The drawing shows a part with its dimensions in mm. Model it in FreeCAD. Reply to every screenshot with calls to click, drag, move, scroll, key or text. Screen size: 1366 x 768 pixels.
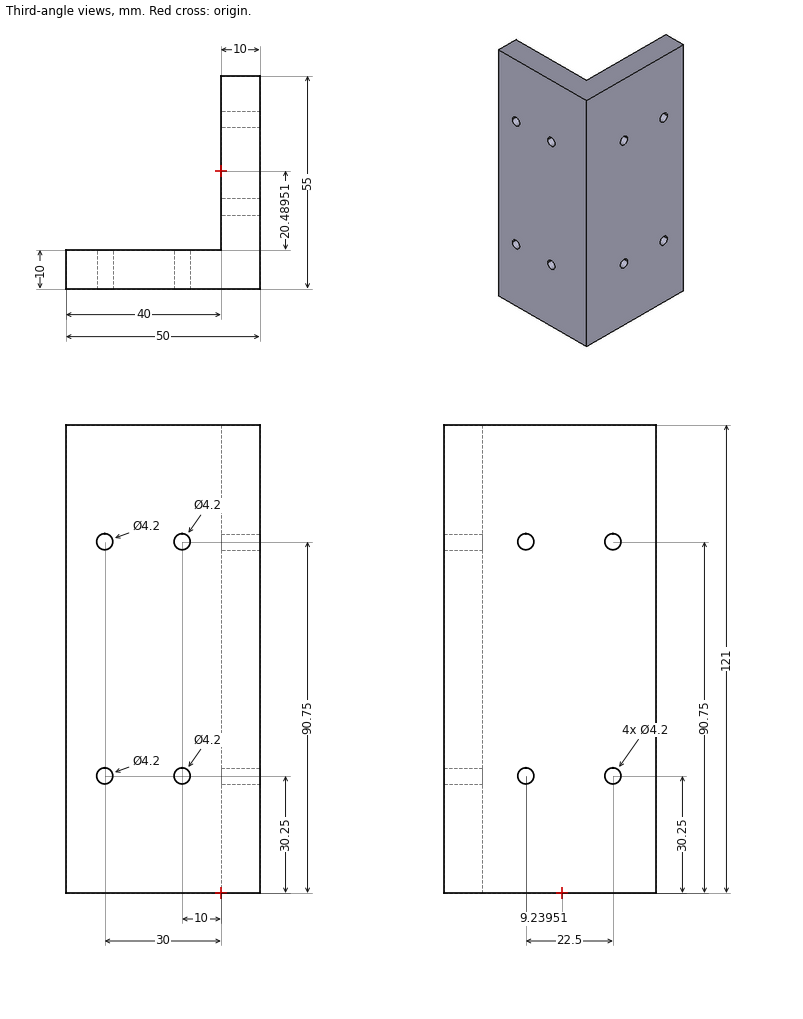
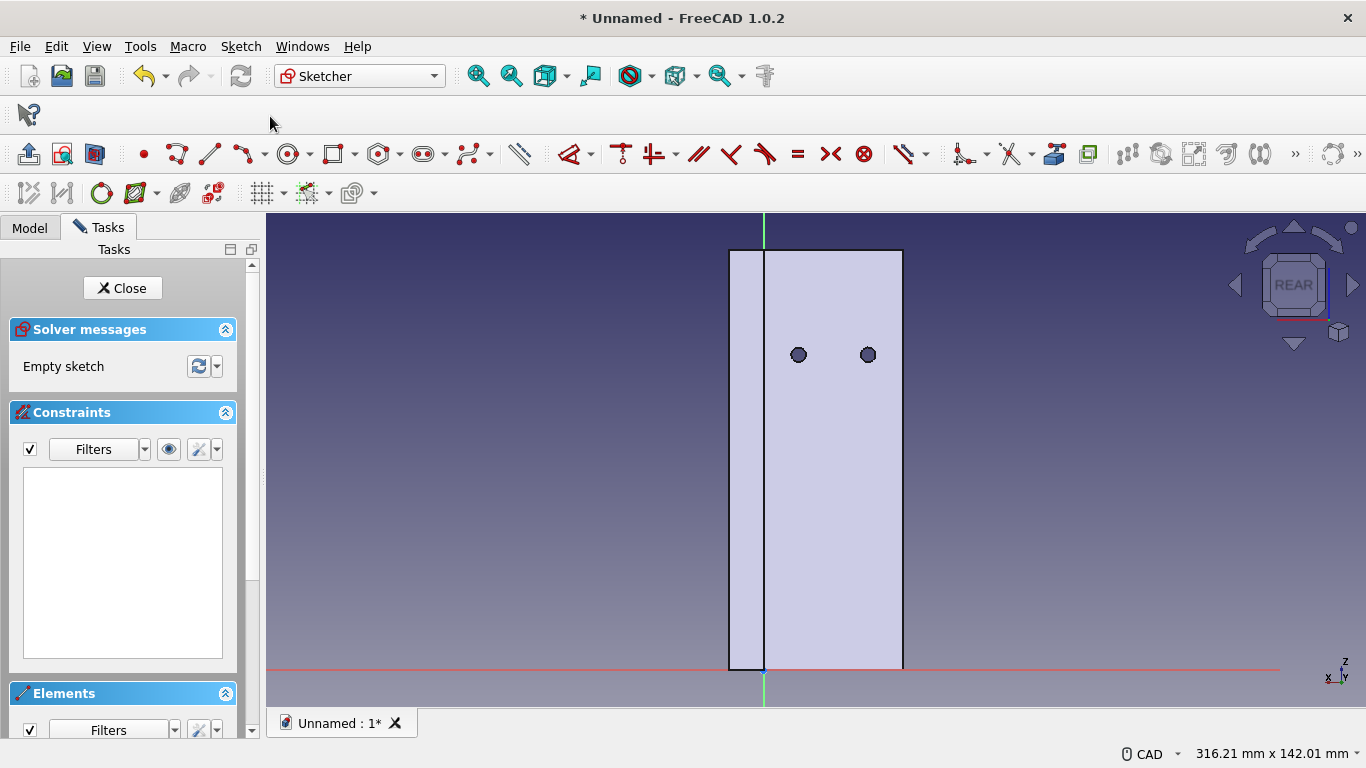
scroll(875, 571, up, 15)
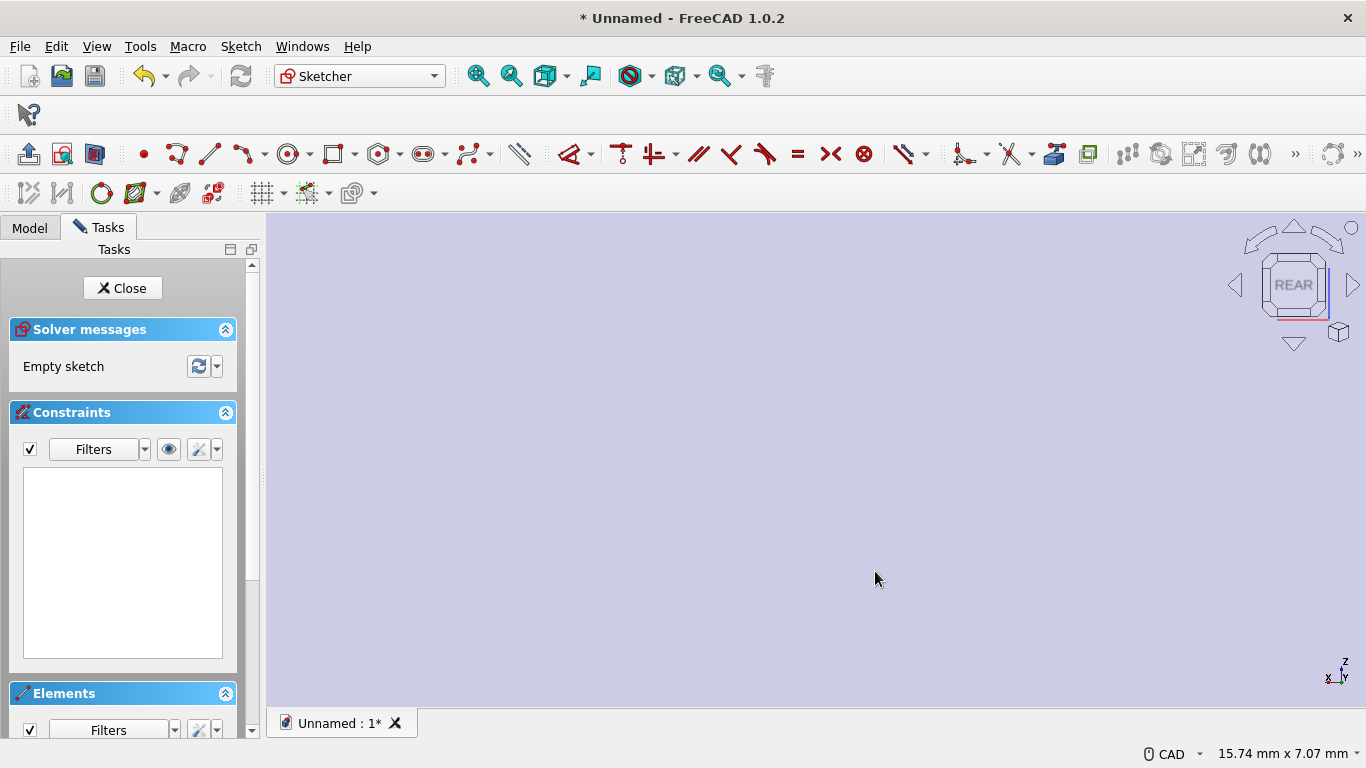
key(g)
key(c)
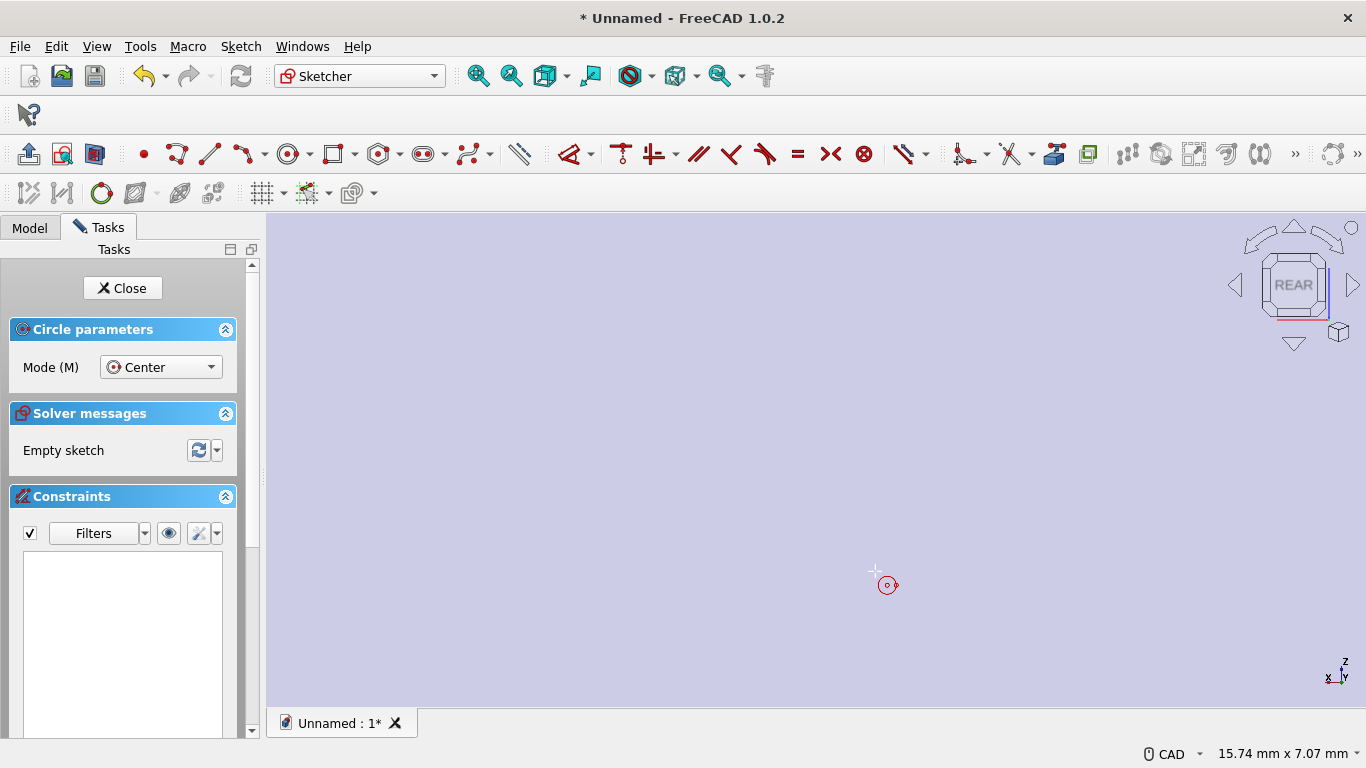
click(727, 441)
move(831, 338)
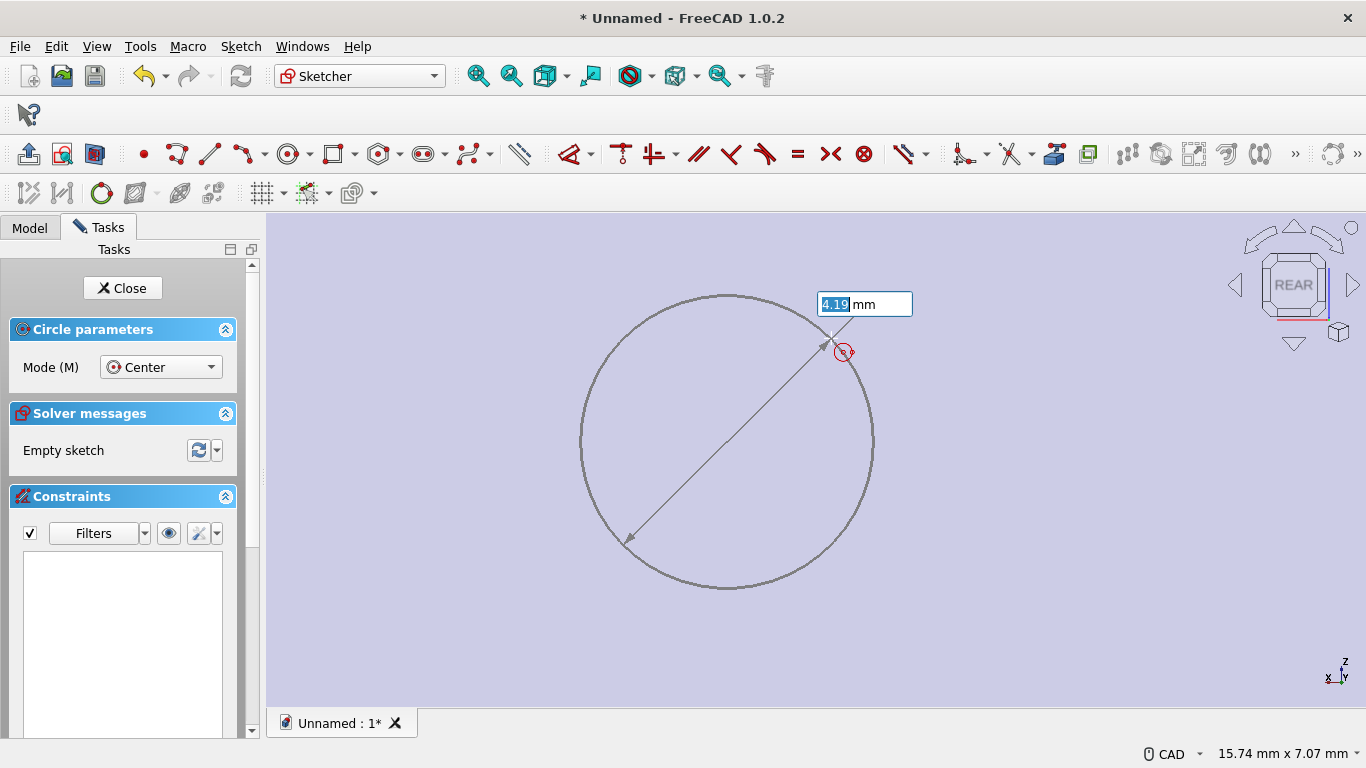
text(4.2)
key(Return)
key(Escape)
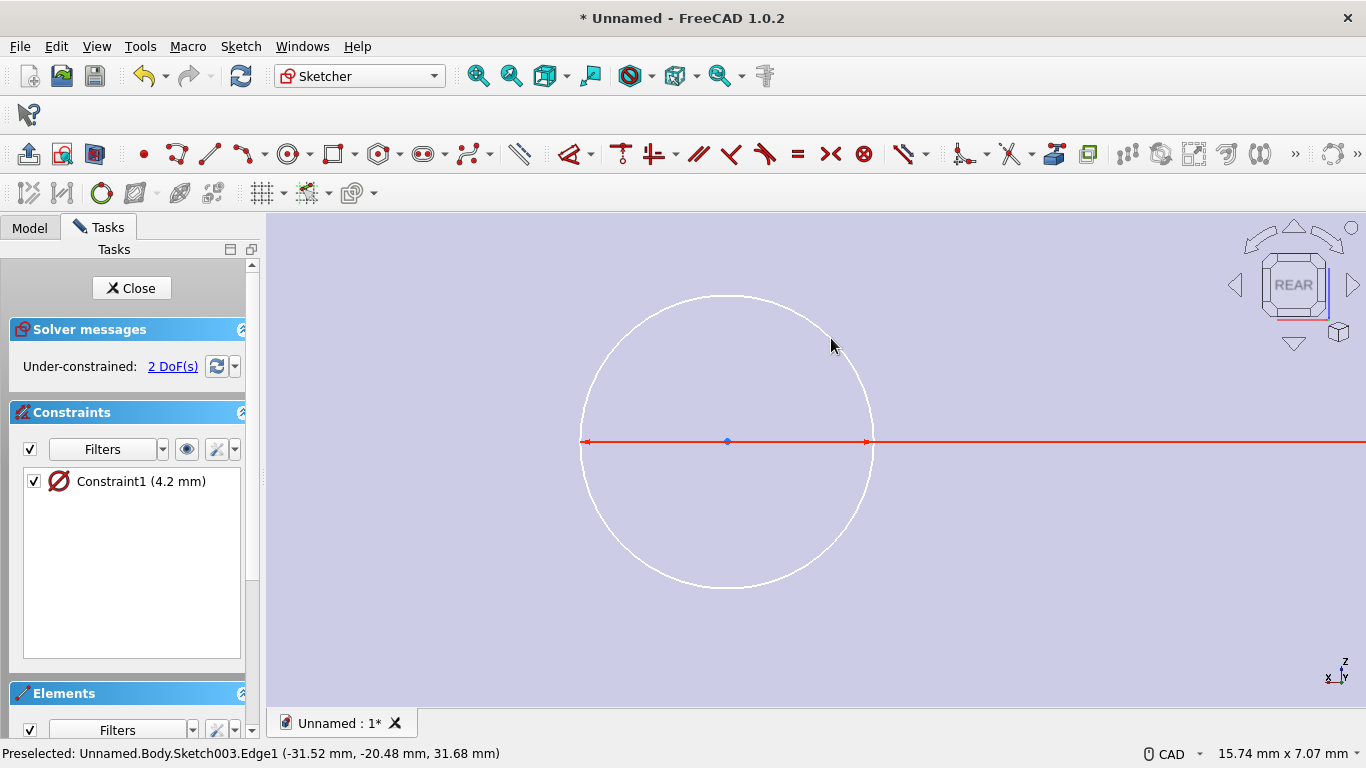
click(568, 154)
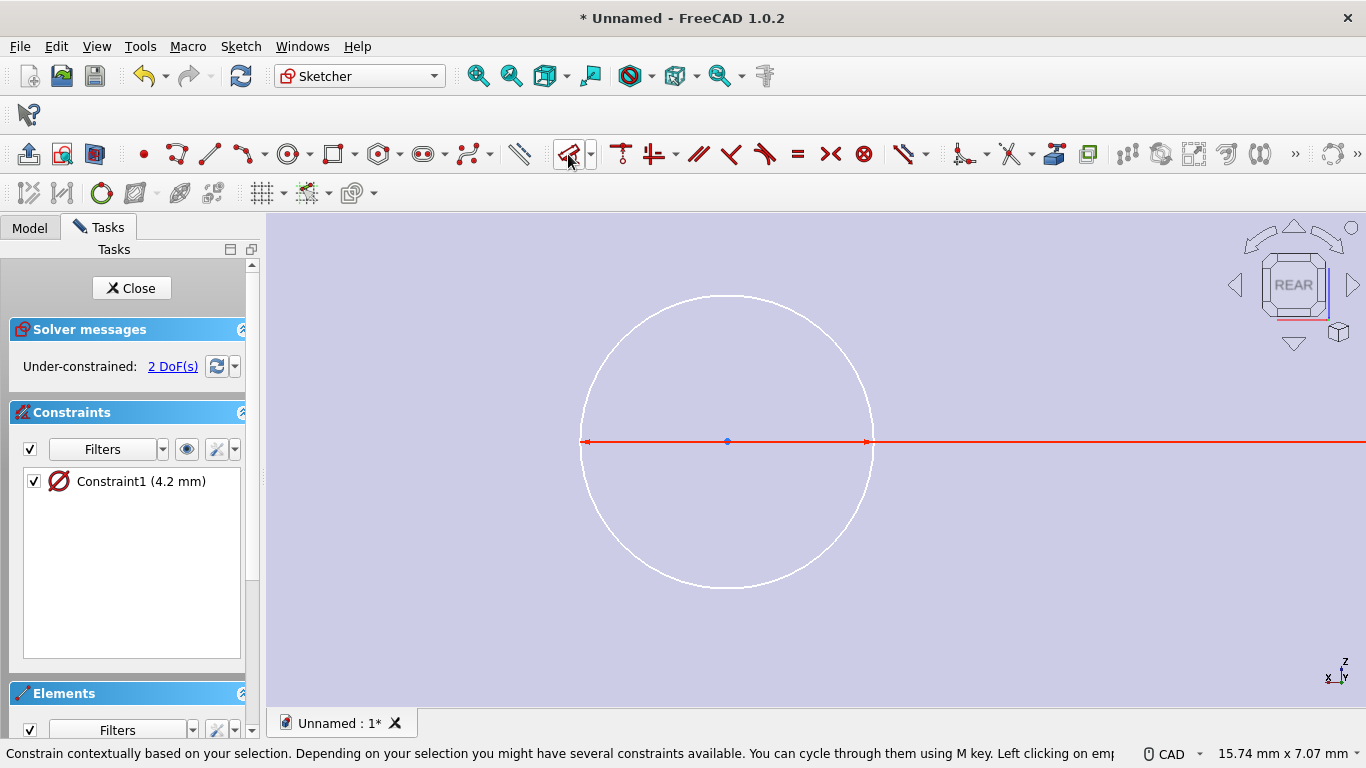
click(727, 442)
click(511, 408)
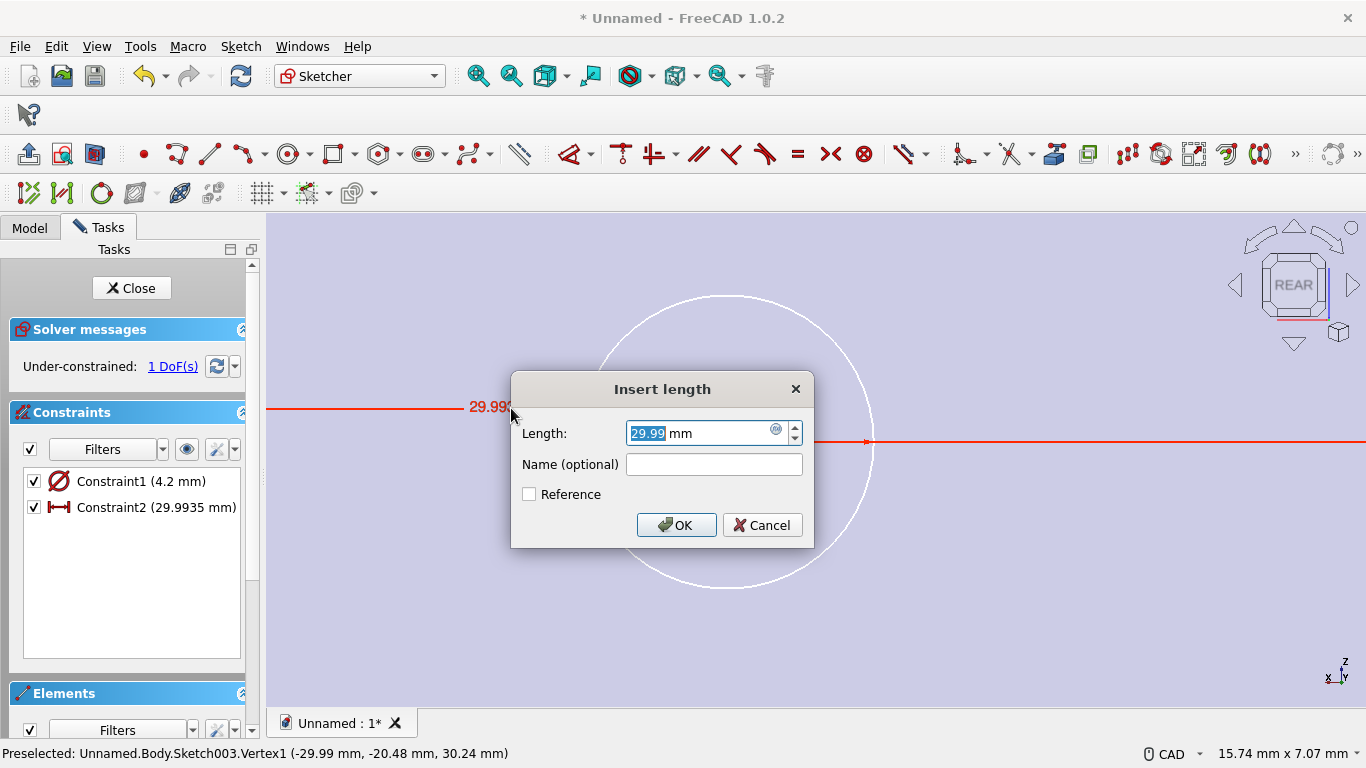
text(30)
key(Return)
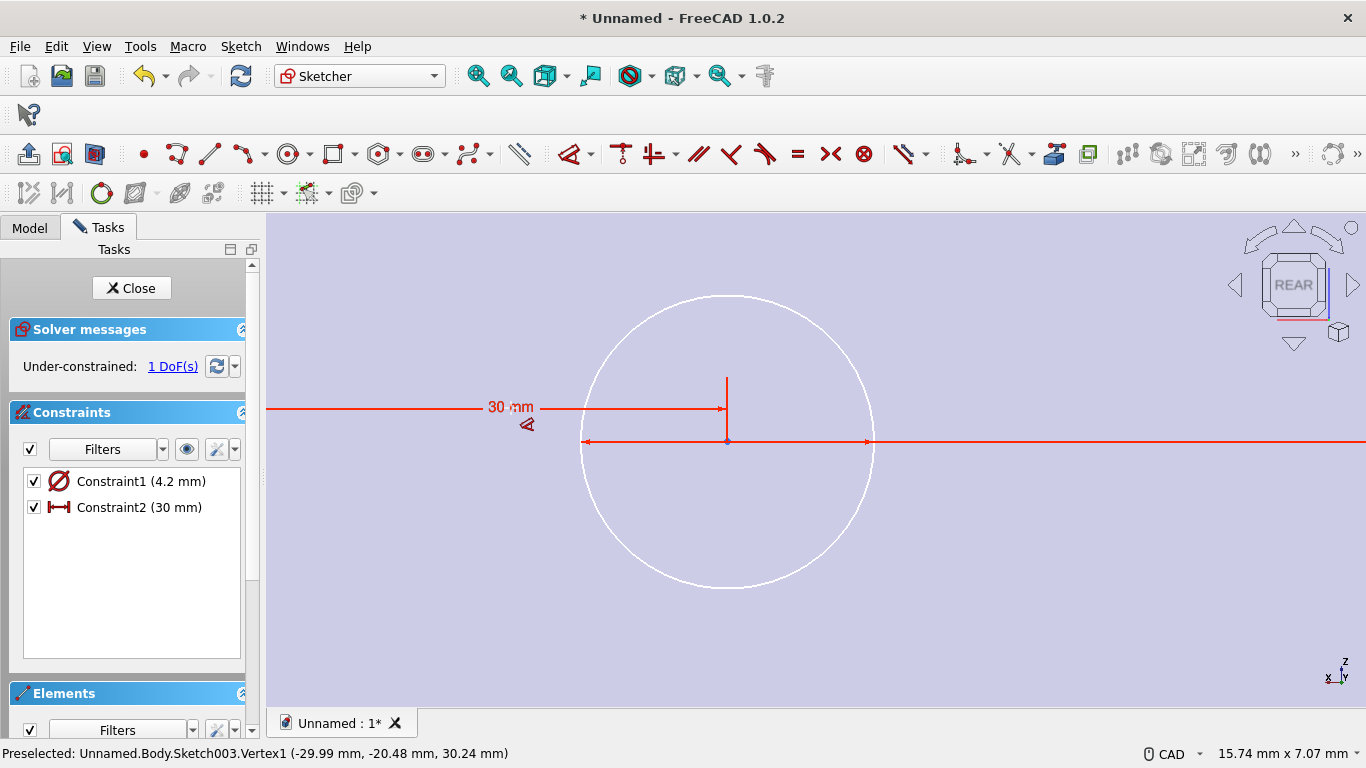
click(727, 442)
click(761, 561)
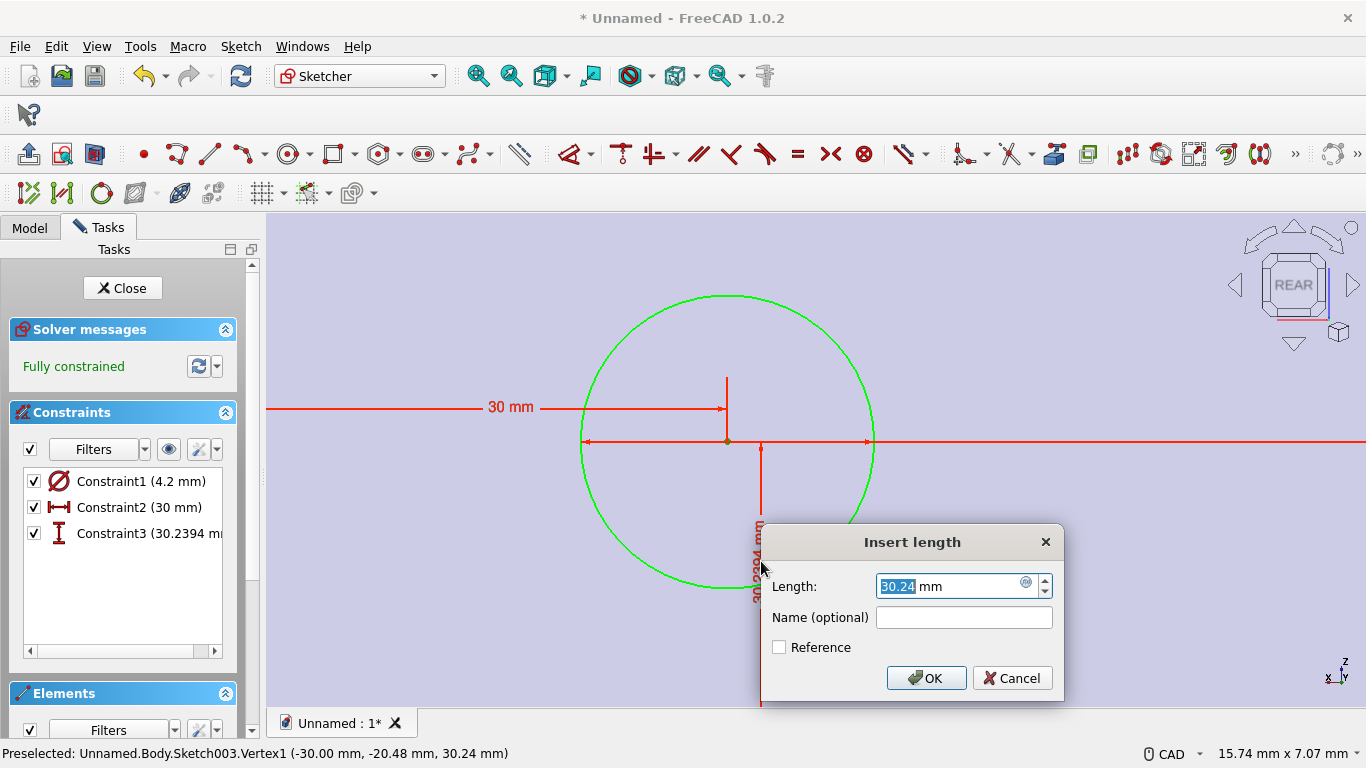
text(30.25)
key(Return)
key(Escape)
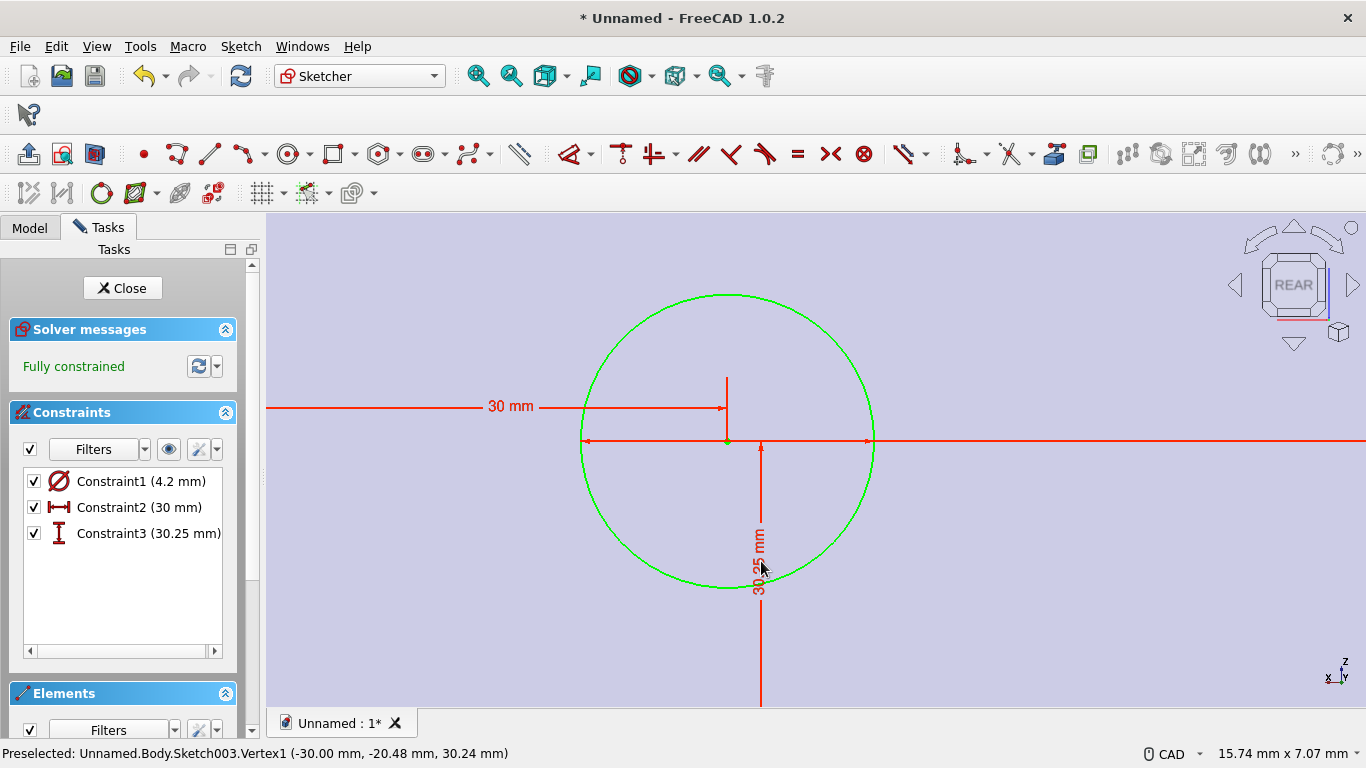
click(123, 288)